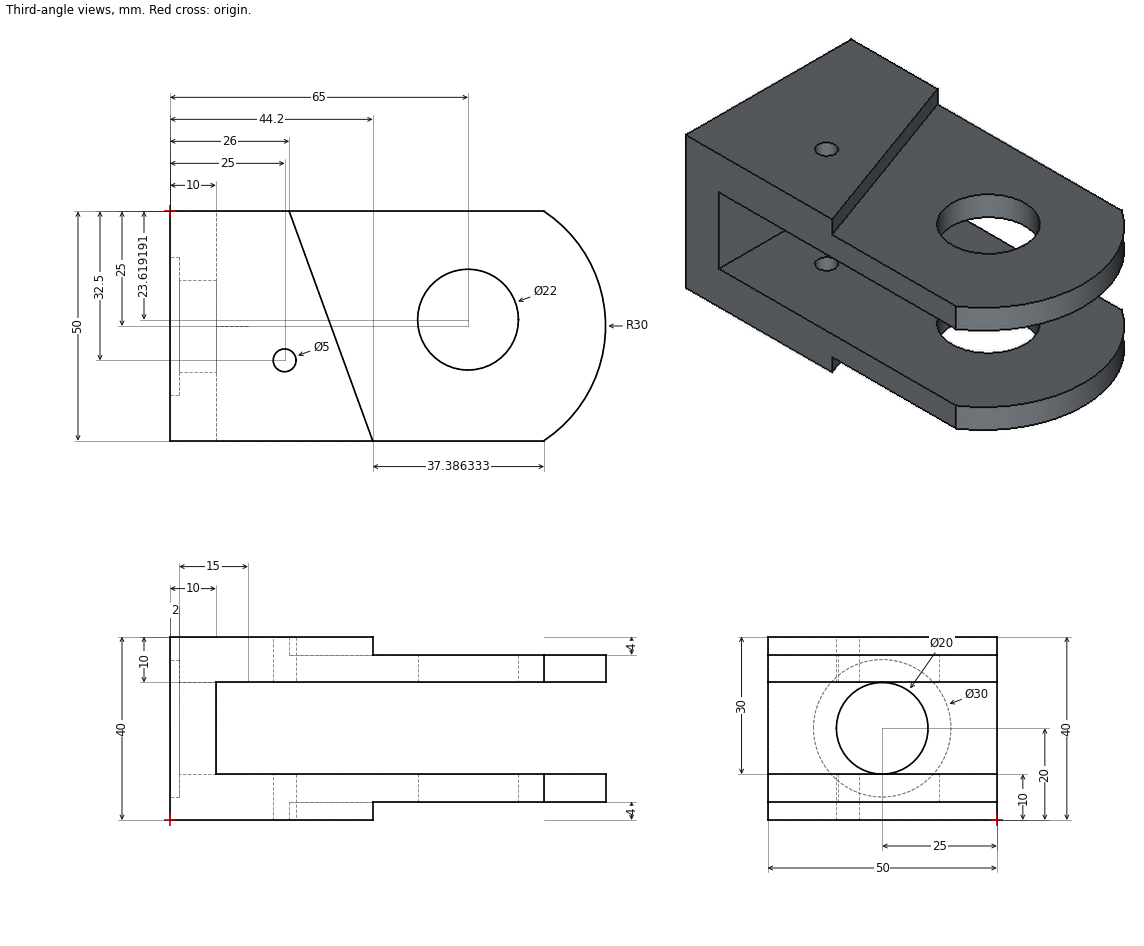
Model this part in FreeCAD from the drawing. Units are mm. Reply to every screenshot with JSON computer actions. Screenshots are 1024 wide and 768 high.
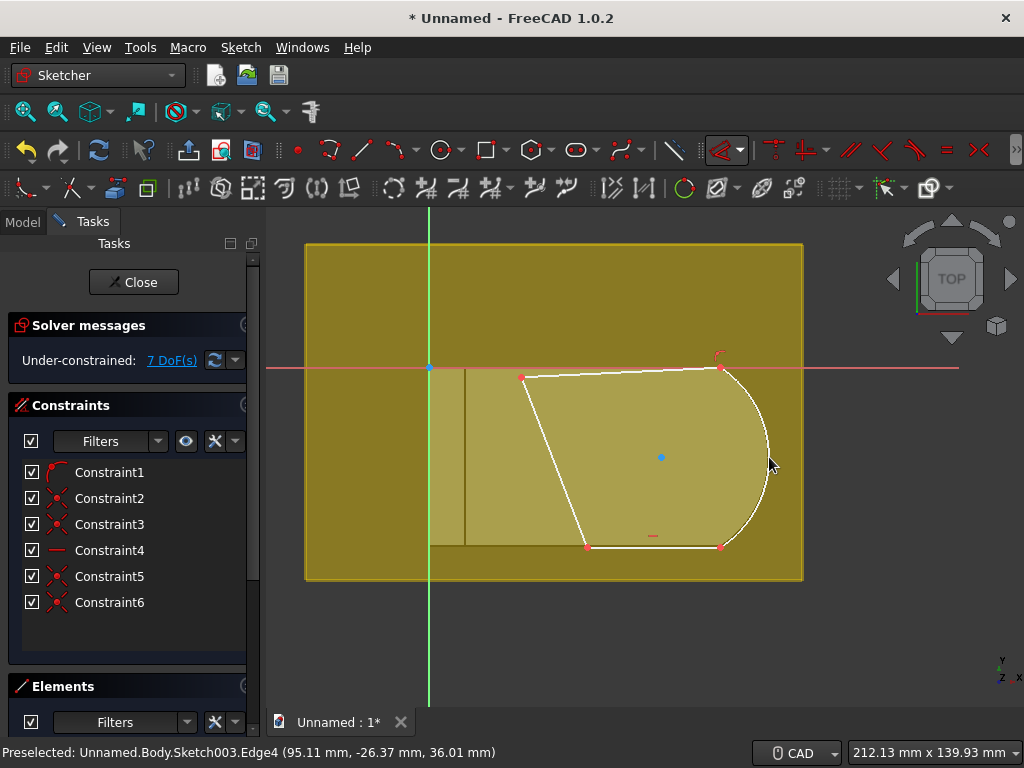
{"action": "left_click", "coordinate": [661, 371]}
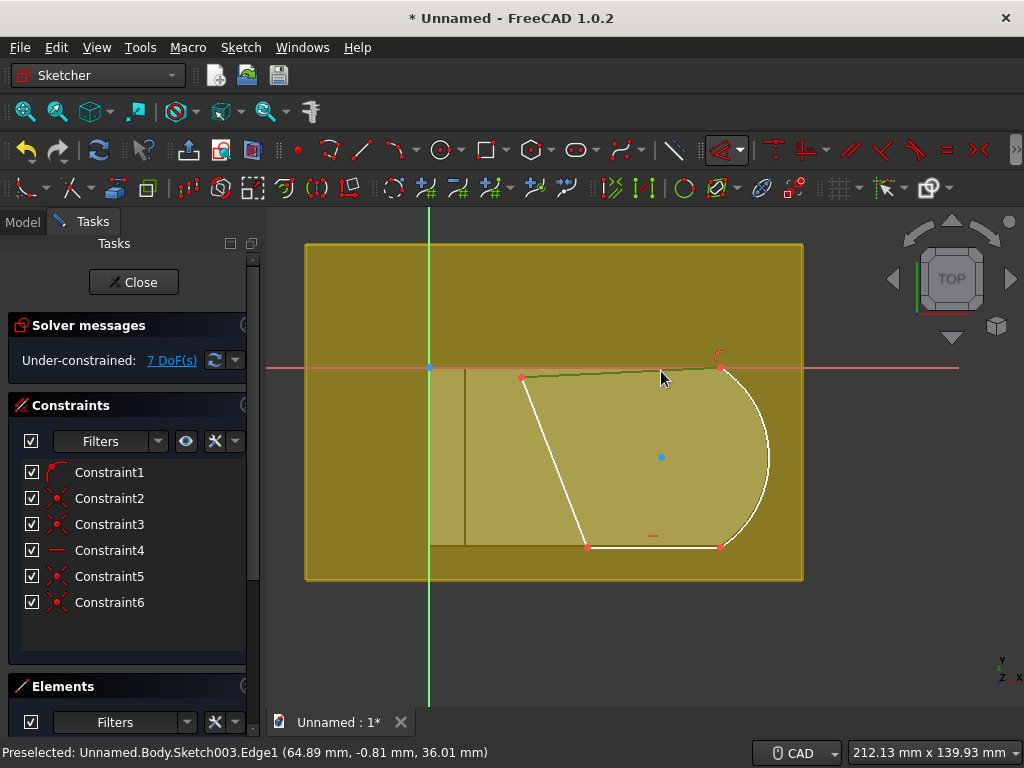
{"action": "key", "text": "h"}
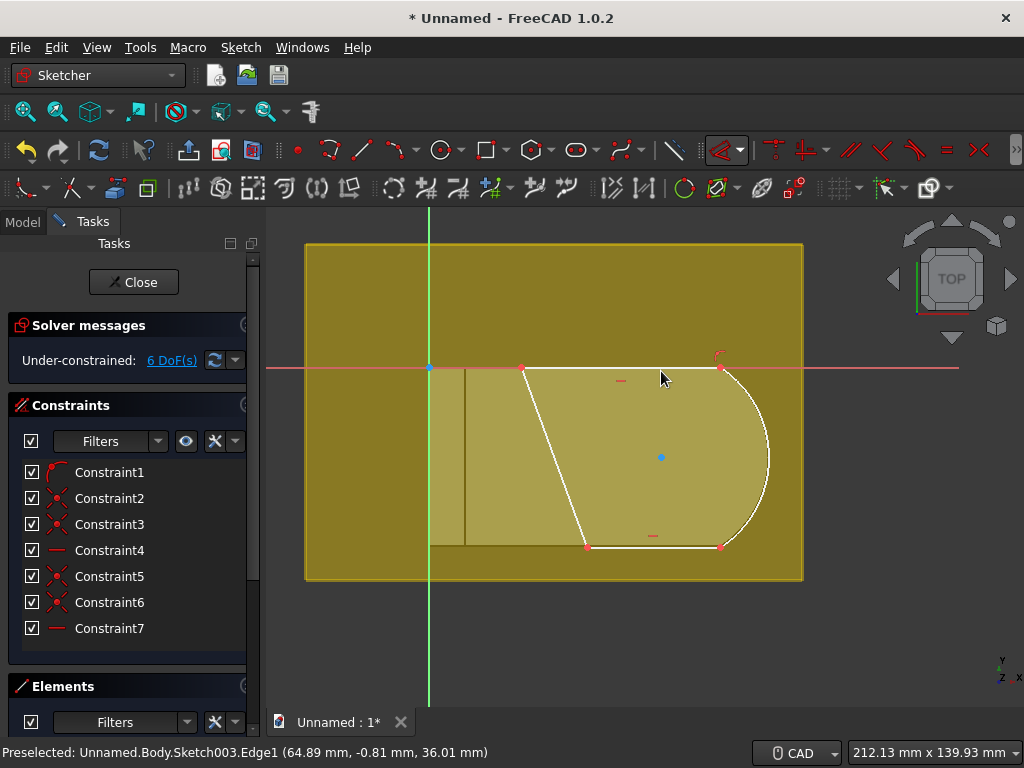
{"action": "left_click", "coordinate": [761, 499]}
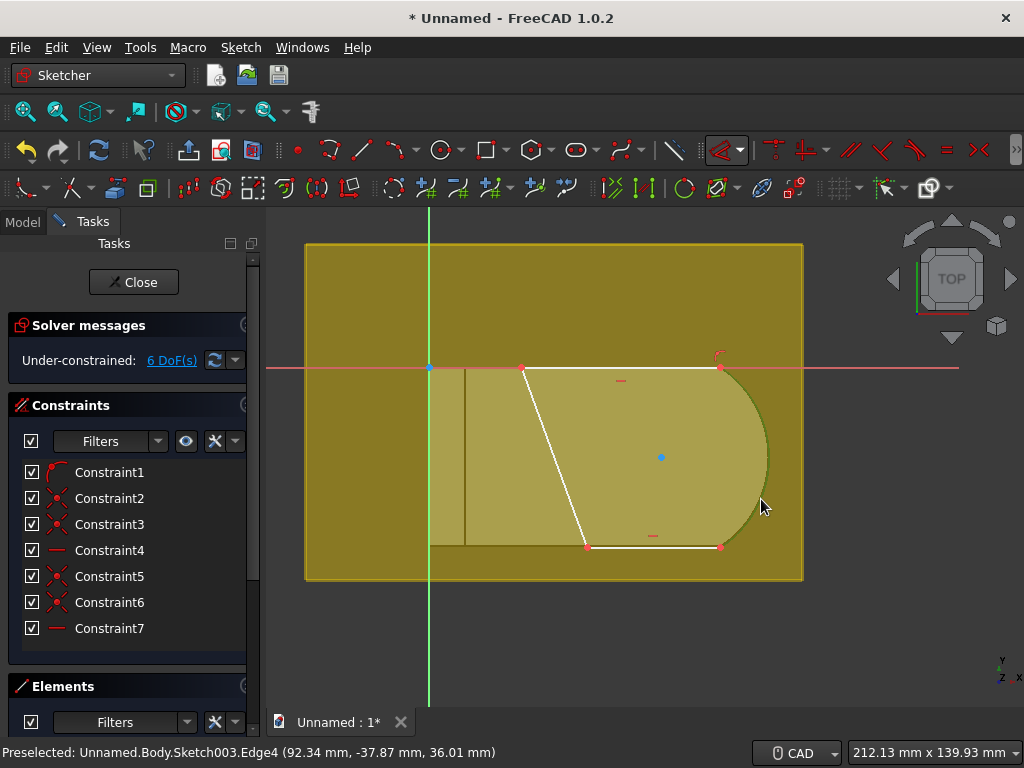
{"action": "left_click", "coordinate": [742, 150]}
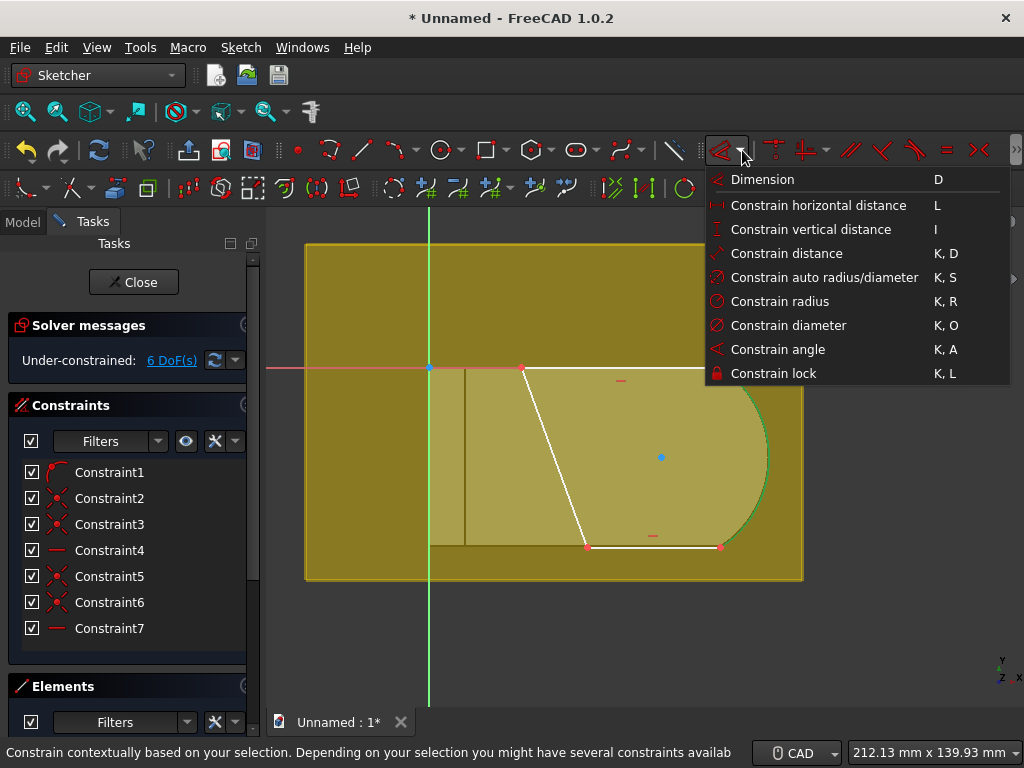
{"action": "left_click", "coordinate": [858, 301]}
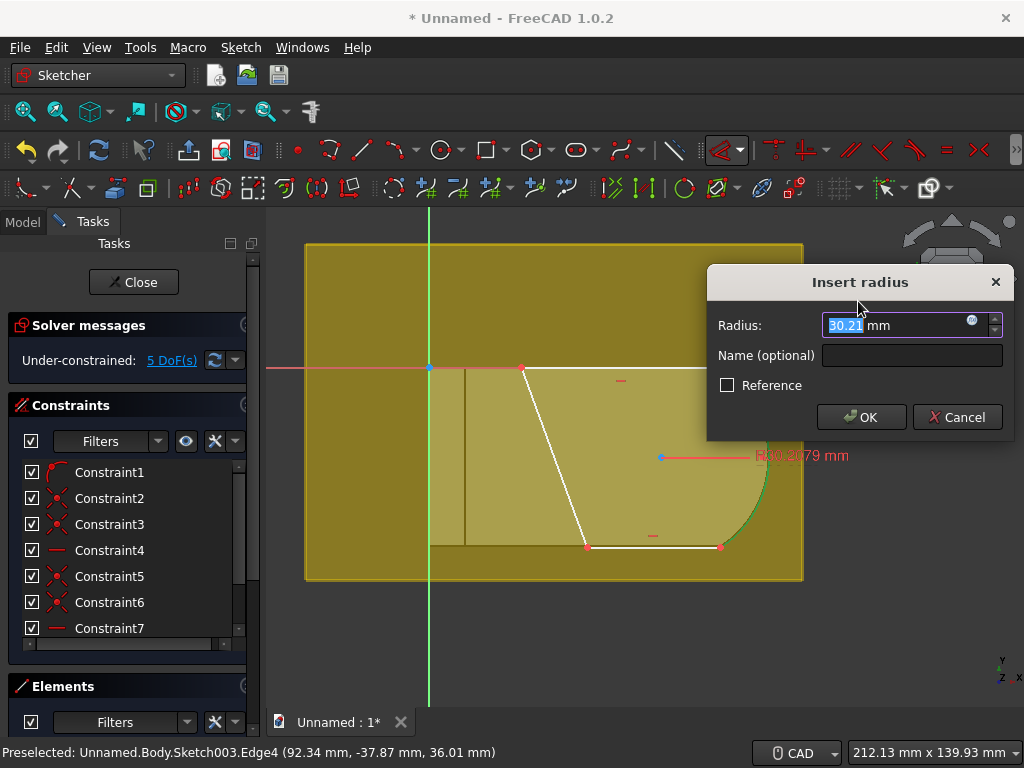
{"action": "type", "text": "30"}
{"action": "key", "text": "Return"}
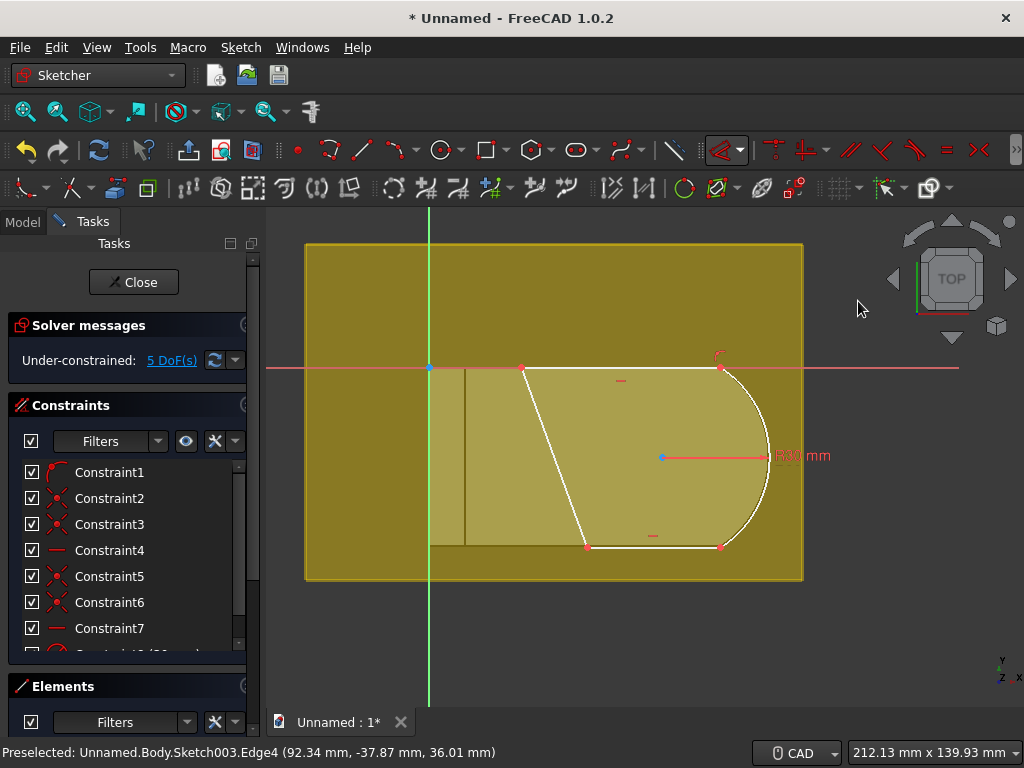
{"action": "left_click", "coordinate": [521, 368]}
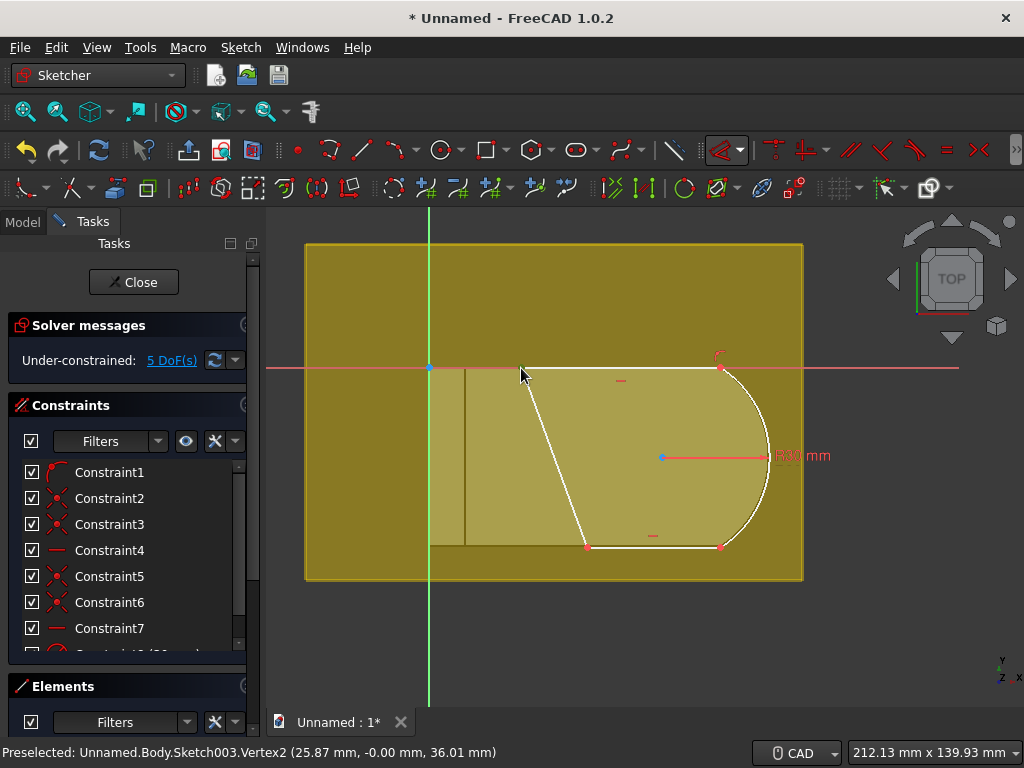
{"action": "left_click", "coordinate": [742, 150]}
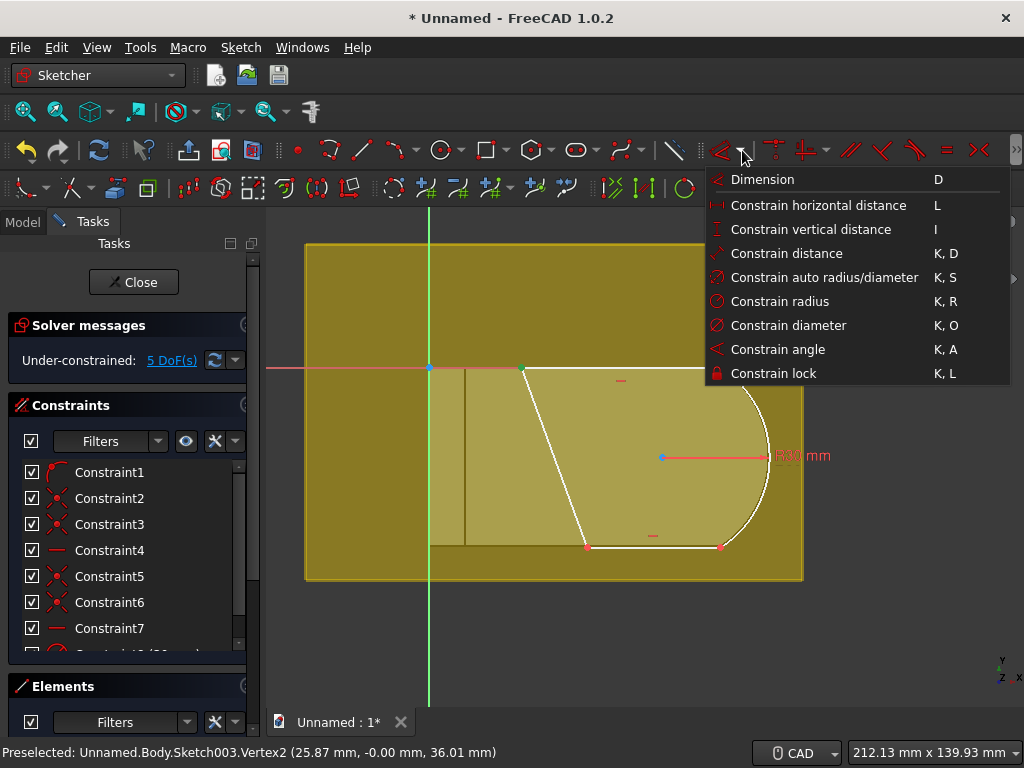
{"action": "left_click", "coordinate": [858, 205]}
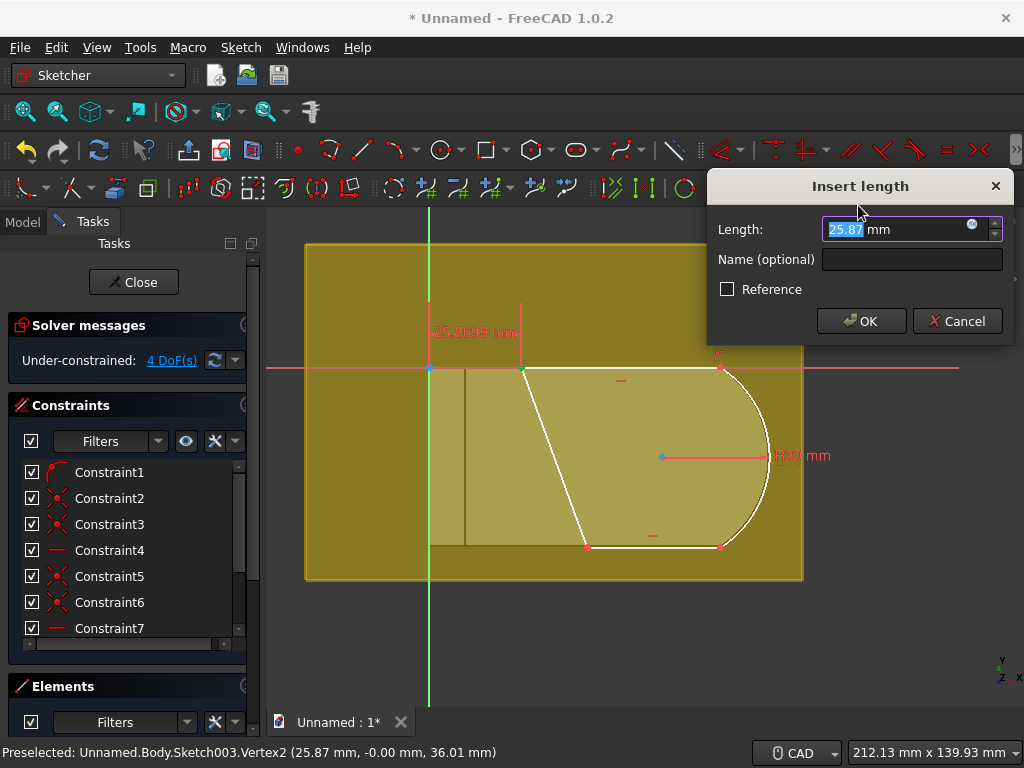
{"action": "type", "text": "26"}
{"action": "key", "text": "Return"}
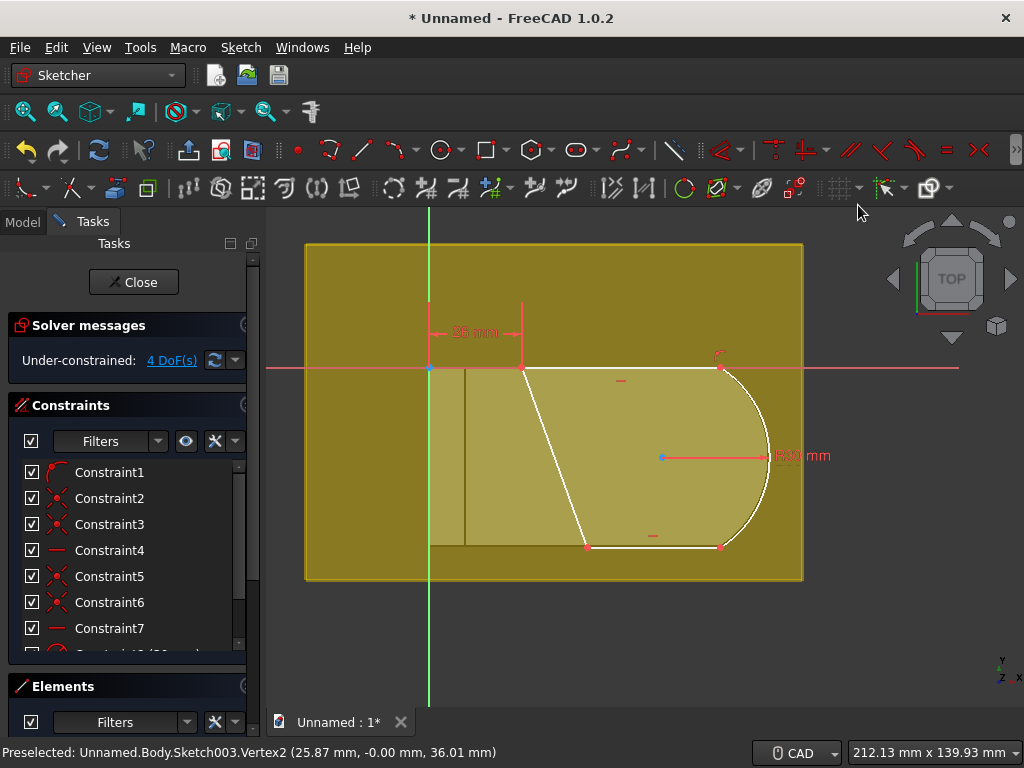
{"action": "left_click", "coordinate": [587, 548]}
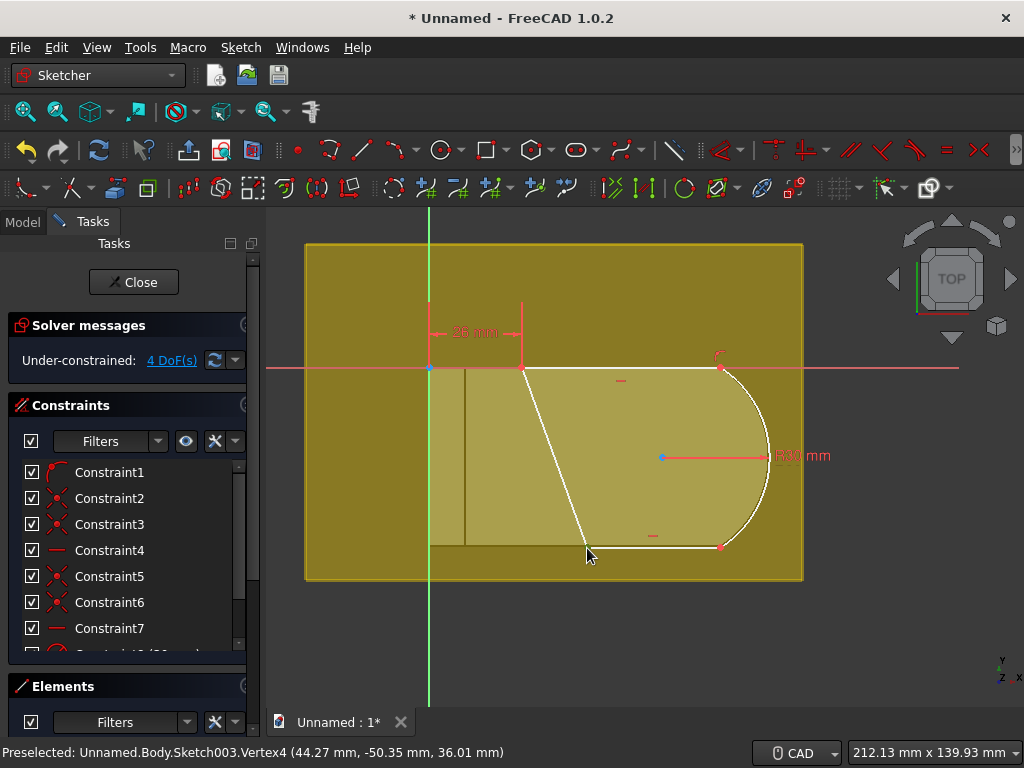
{"action": "key", "text": "i"}